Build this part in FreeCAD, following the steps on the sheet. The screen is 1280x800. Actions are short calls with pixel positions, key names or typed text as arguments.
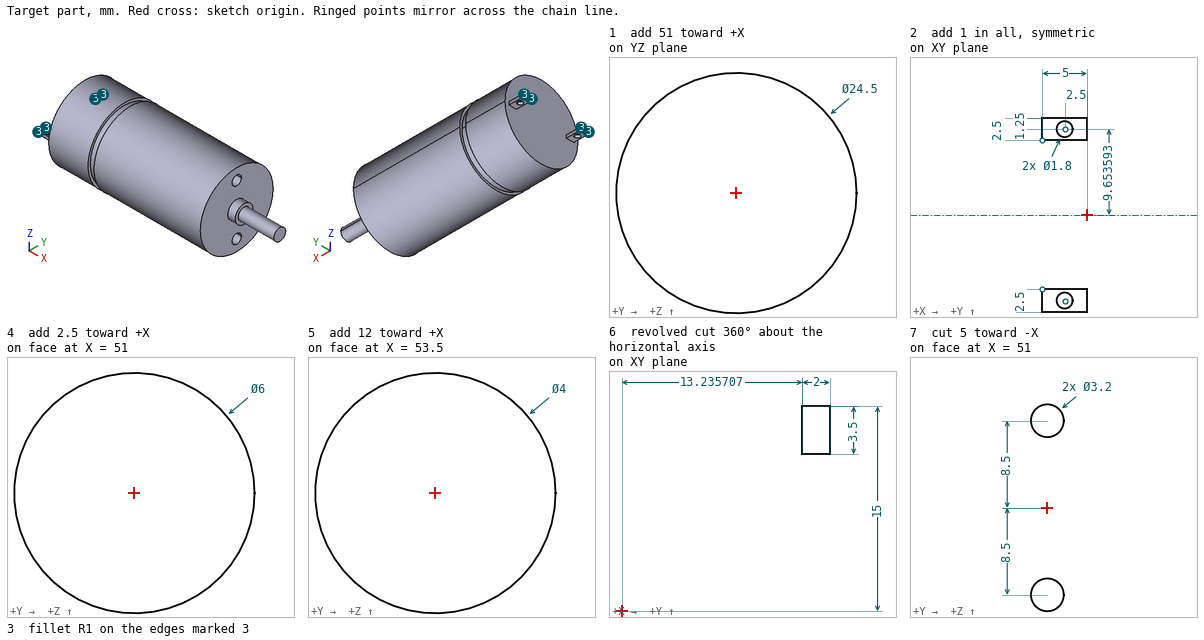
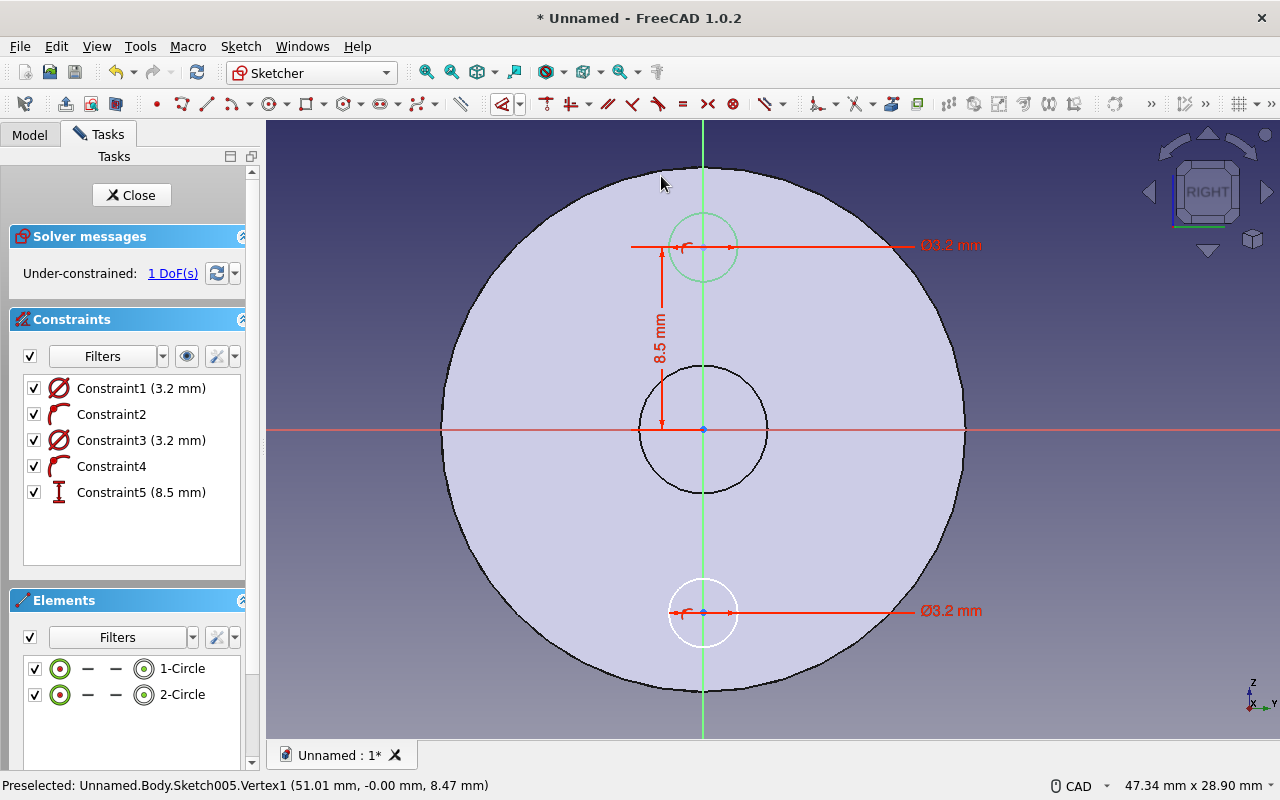
click(703, 613)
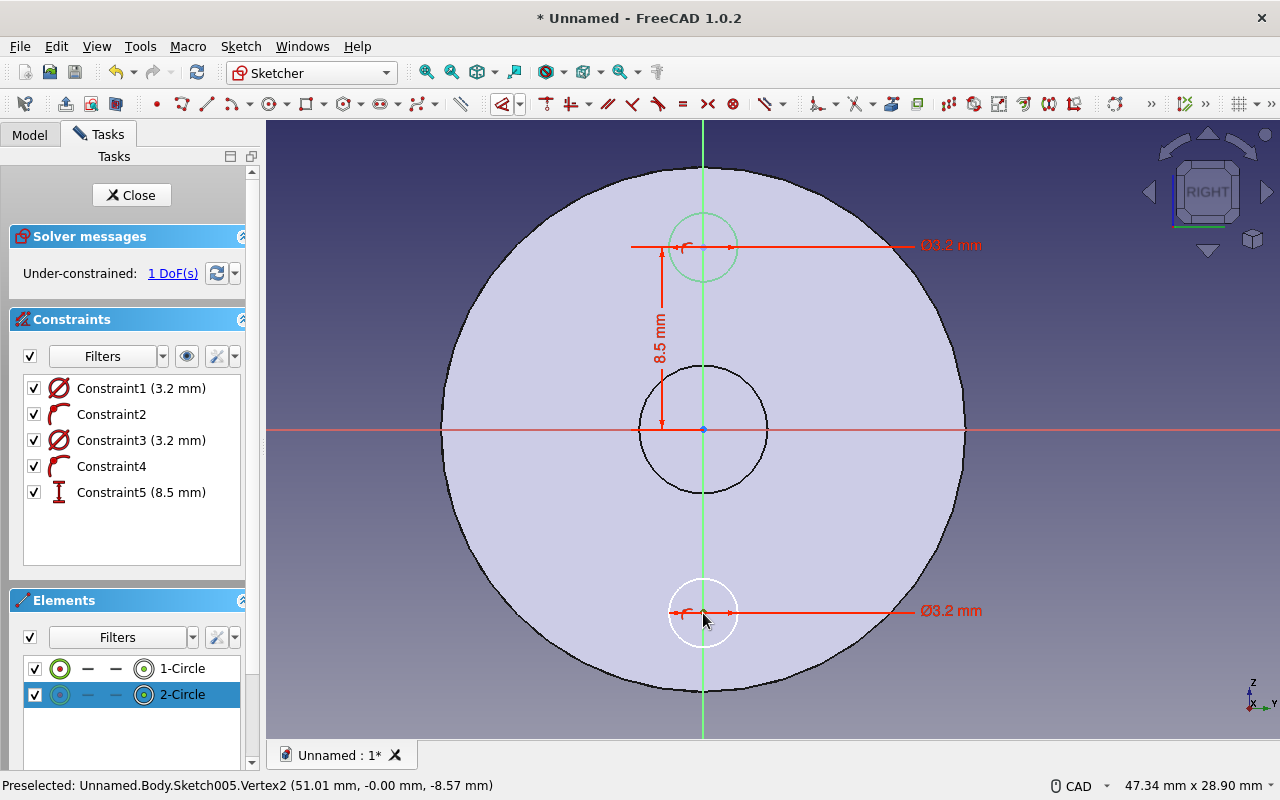
key(i)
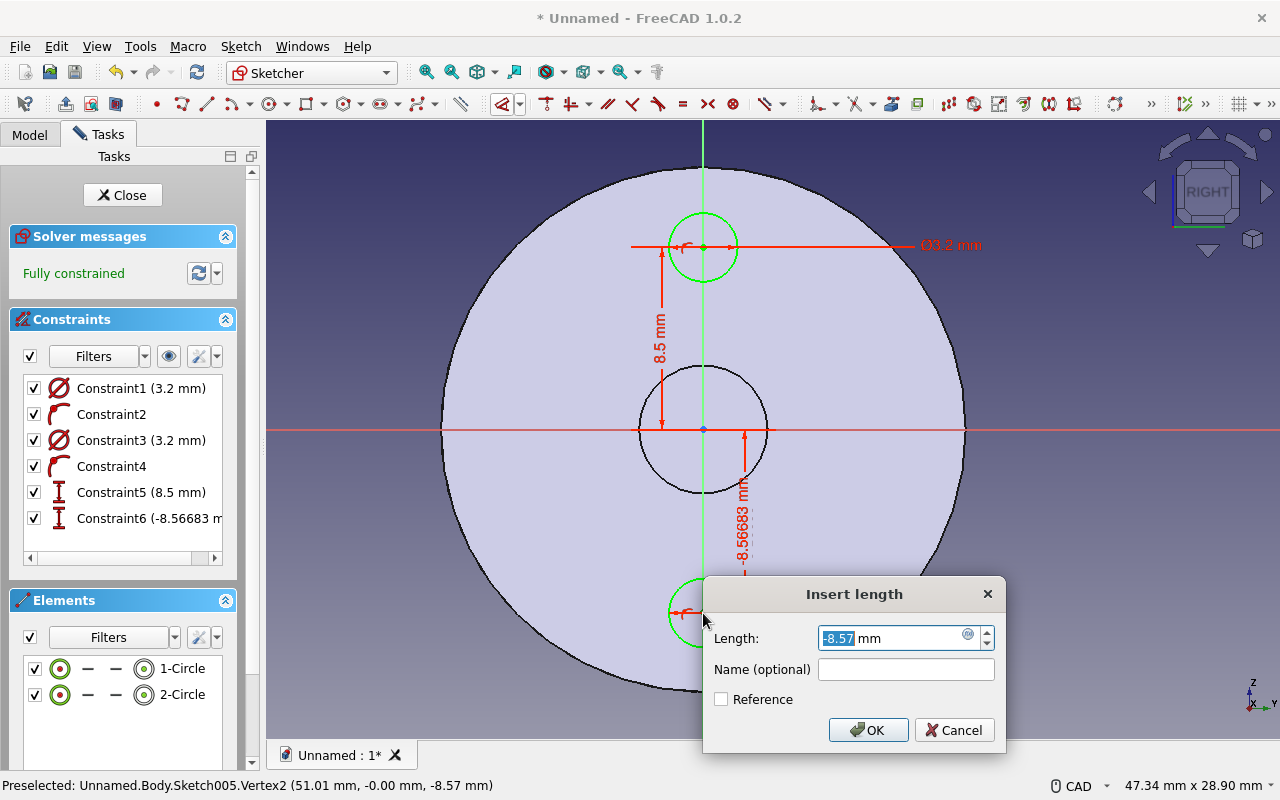
text(-8.5)
key(Return)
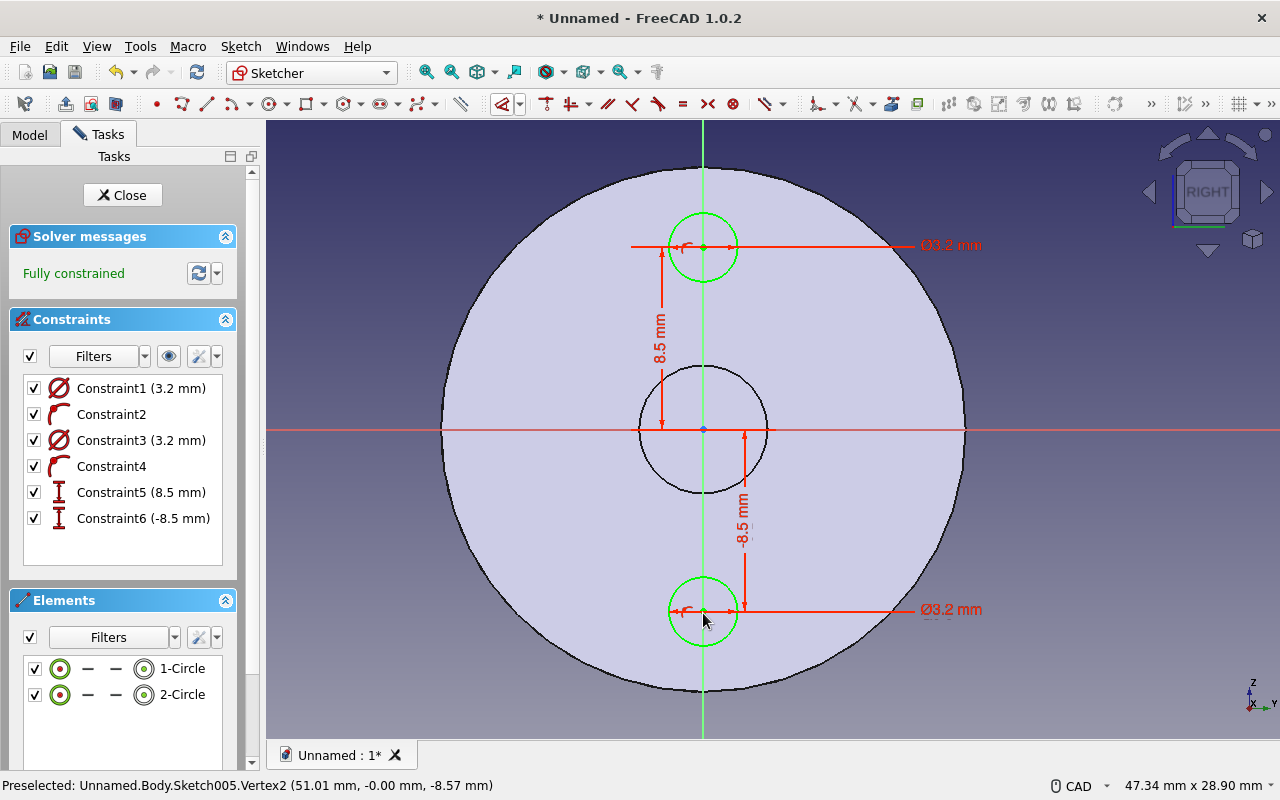
click(123, 195)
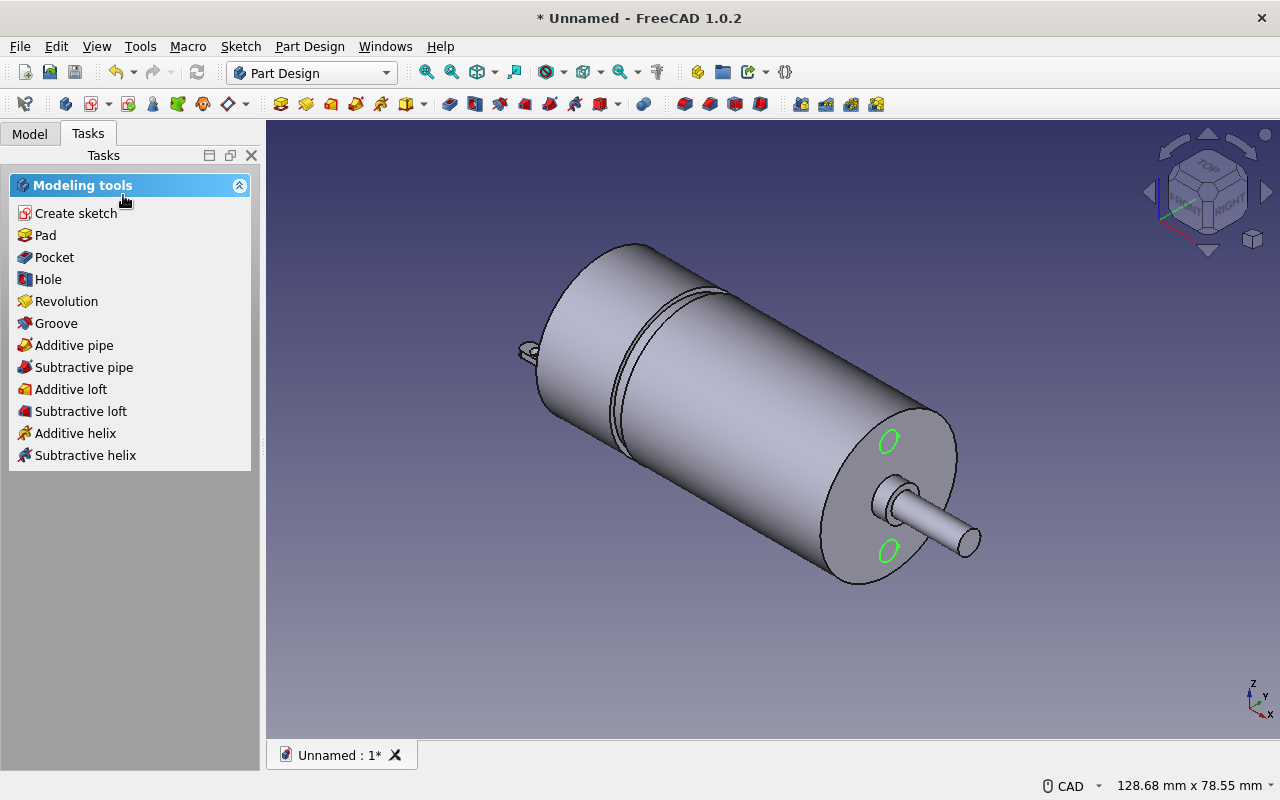
click(450, 104)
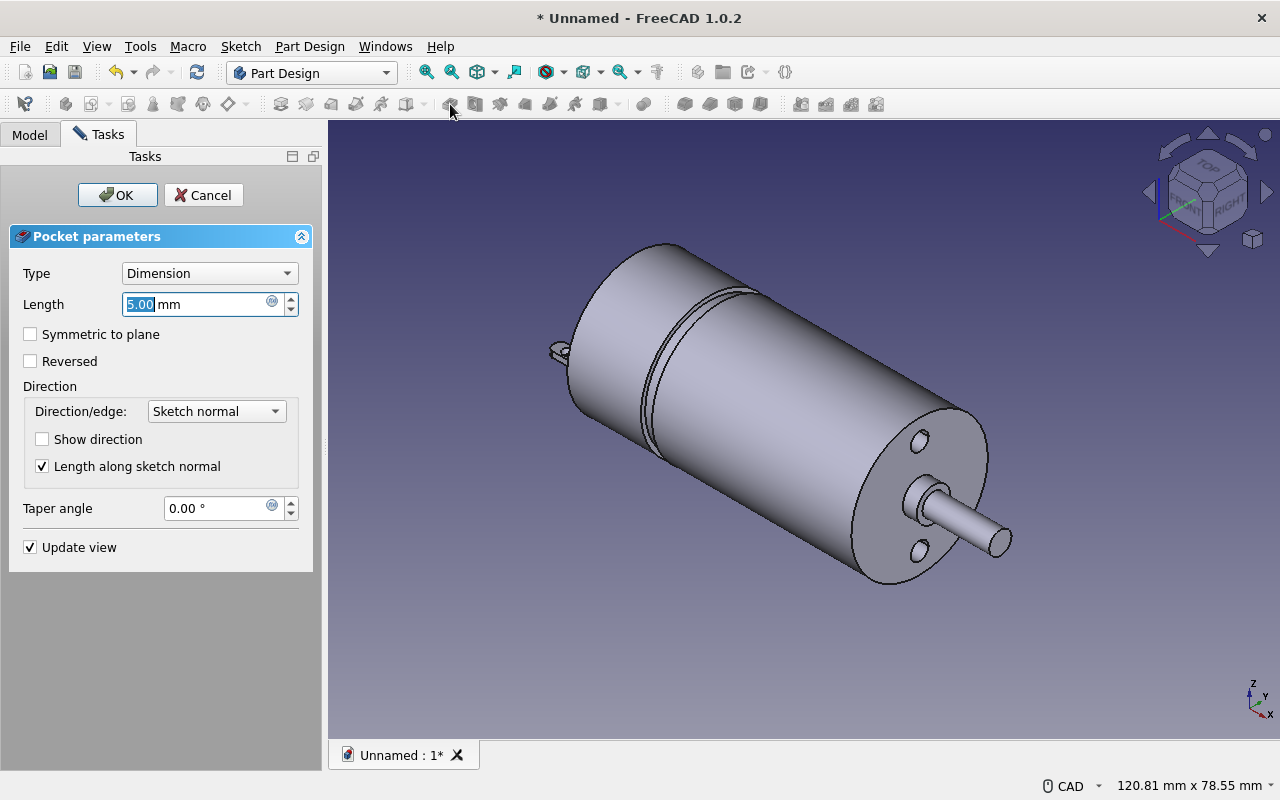
text(5)
key(Tab)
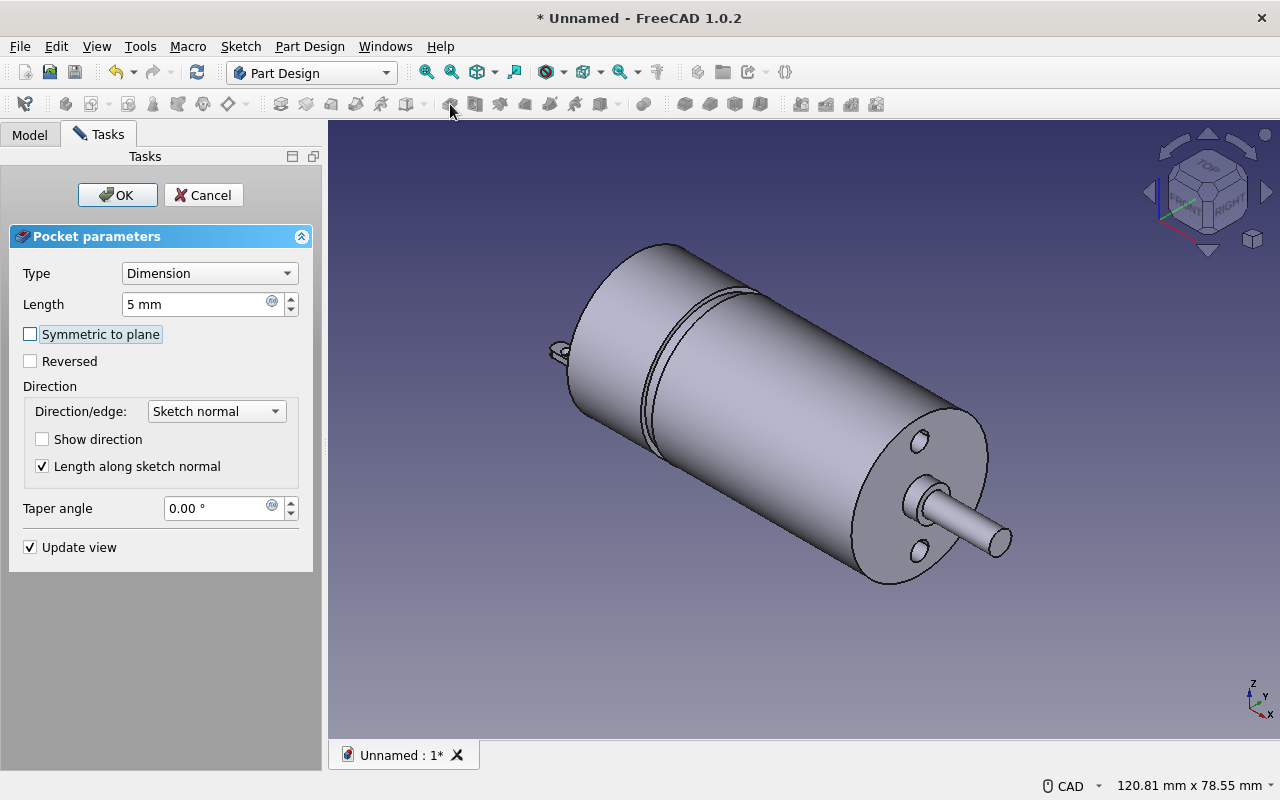
click(118, 195)